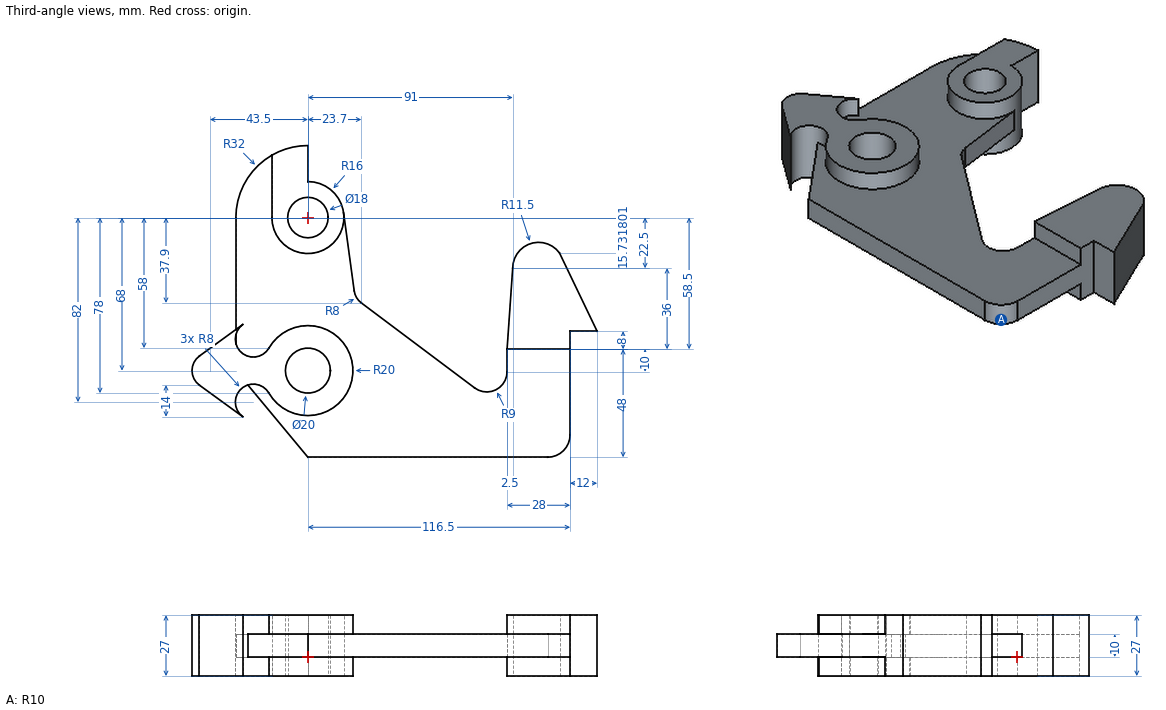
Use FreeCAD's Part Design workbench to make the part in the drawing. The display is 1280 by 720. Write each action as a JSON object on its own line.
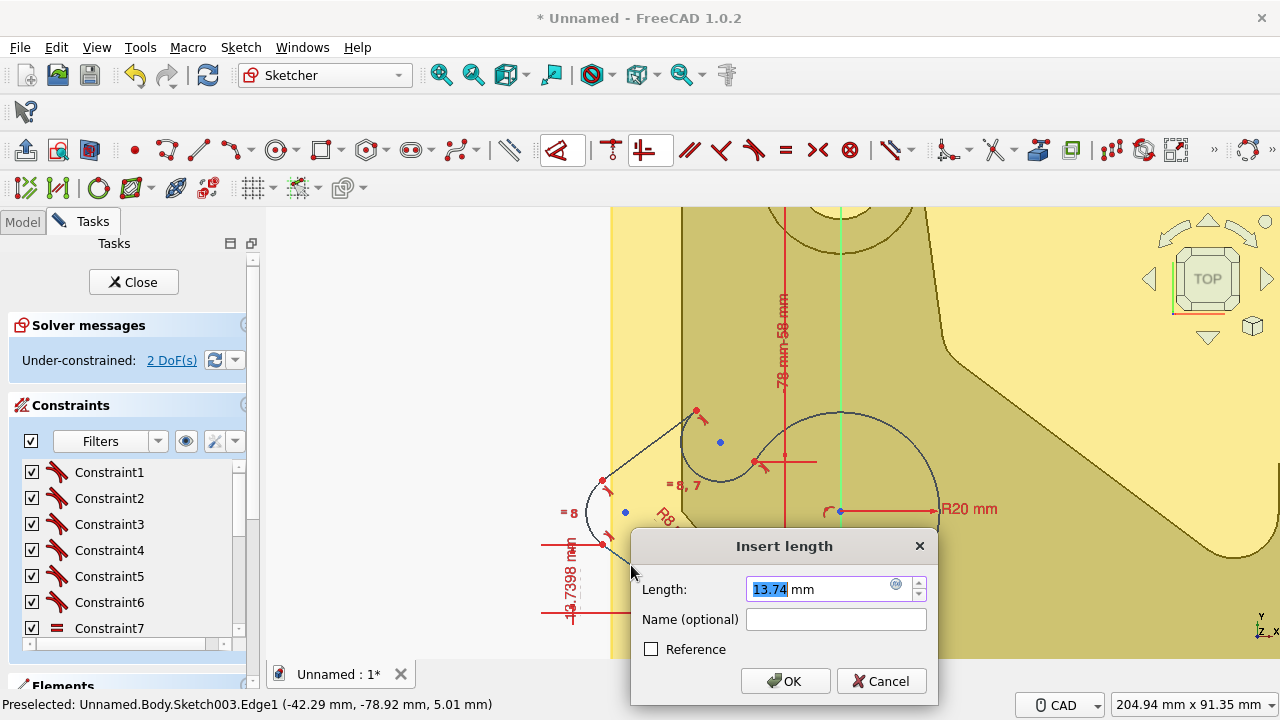
{"action": "type", "text": "14"}
{"action": "key", "text": "Return"}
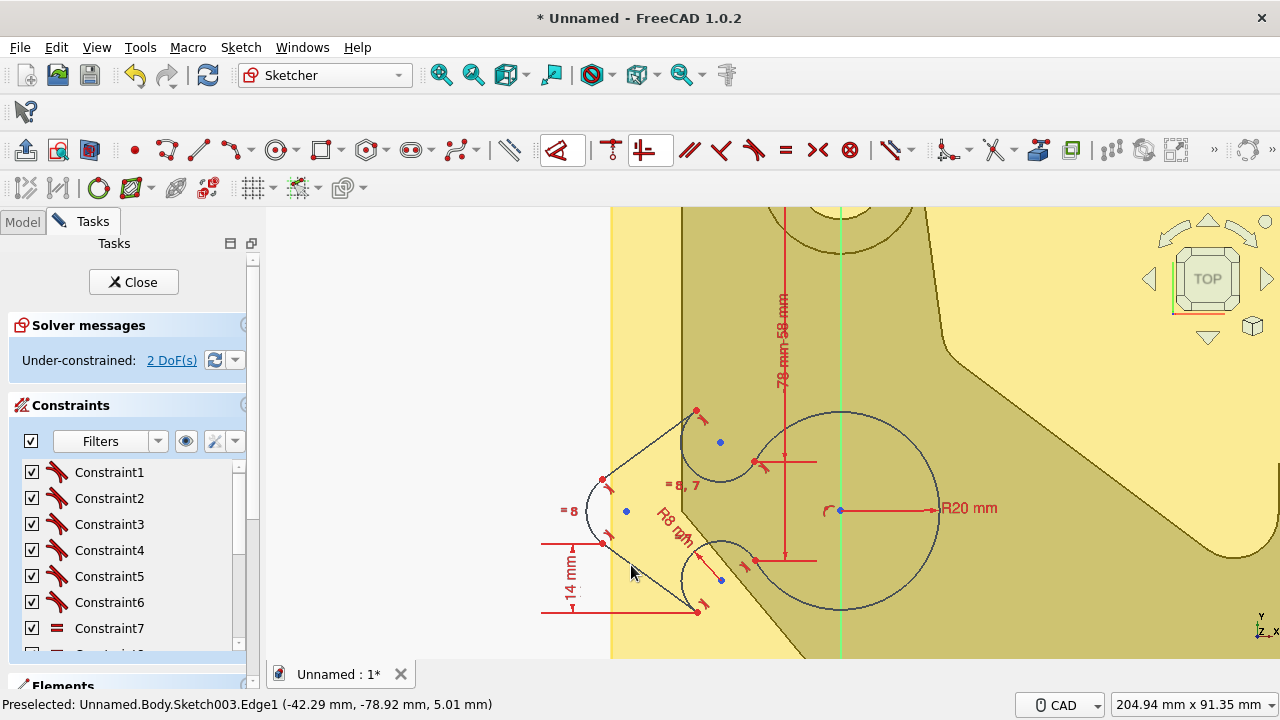
{"action": "left_click", "coordinate": [721, 581]}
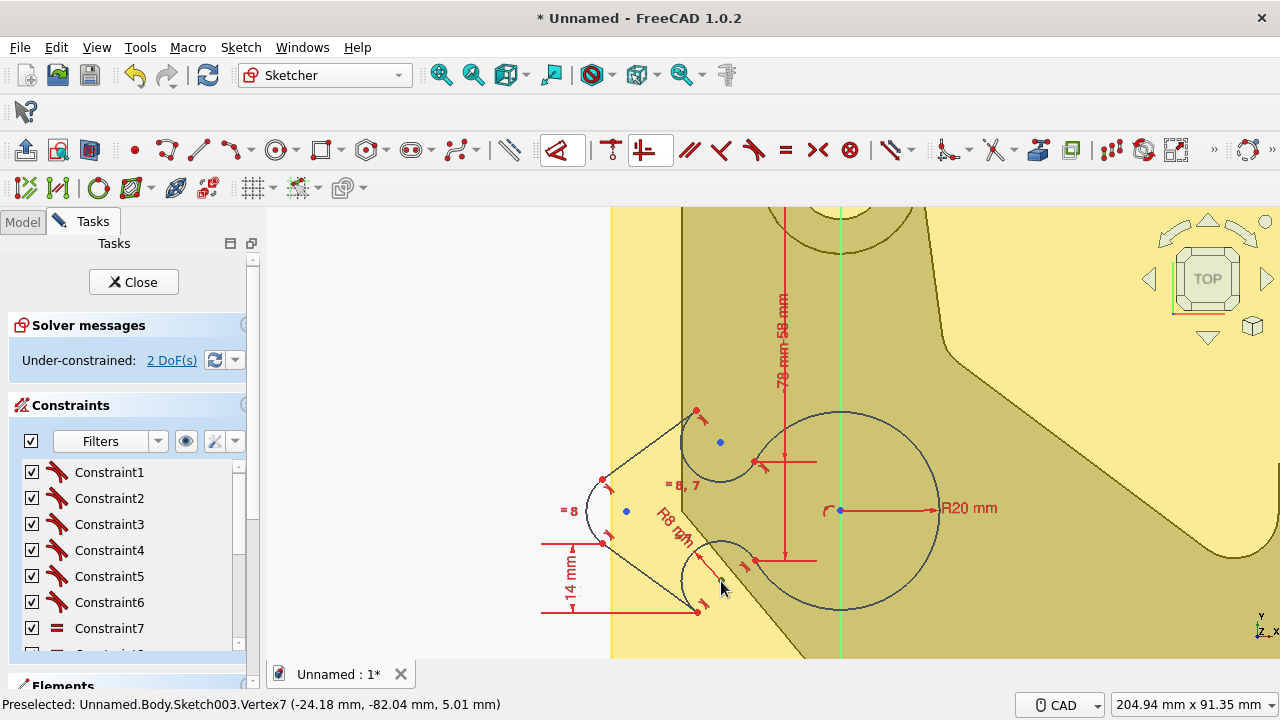
{"action": "left_click", "coordinate": [580, 150]}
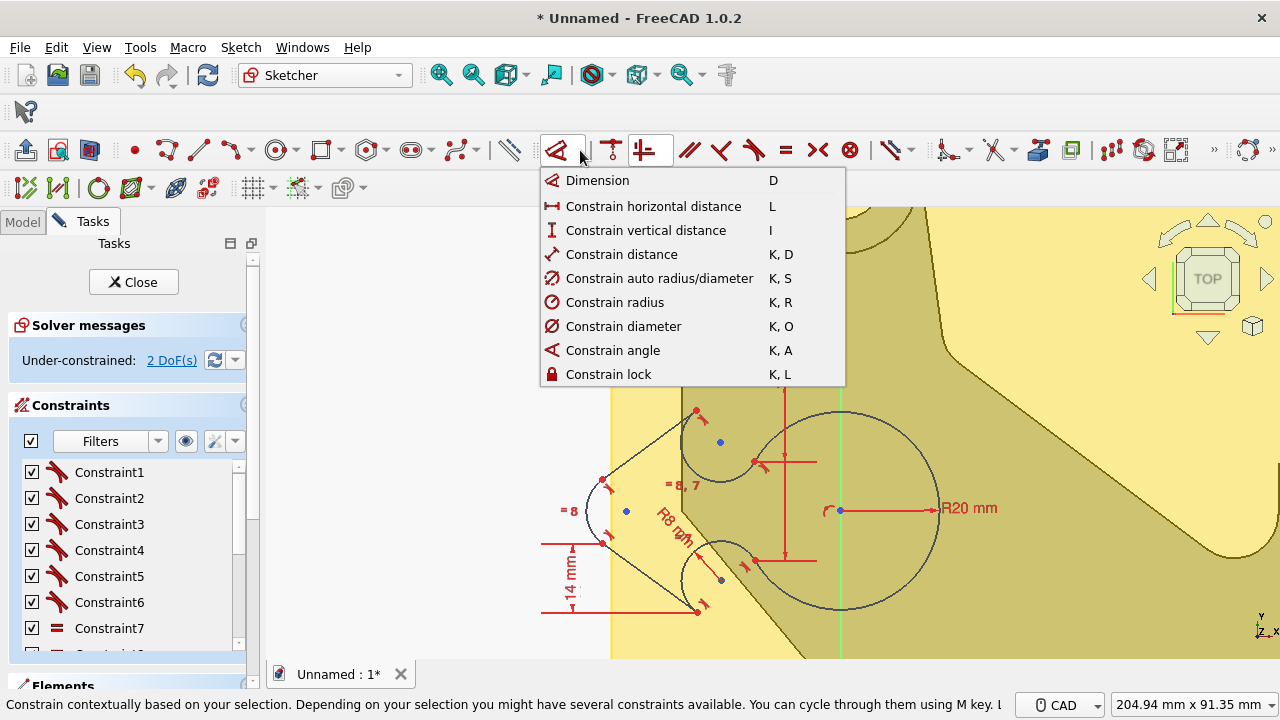
{"action": "left_click", "coordinate": [693, 230]}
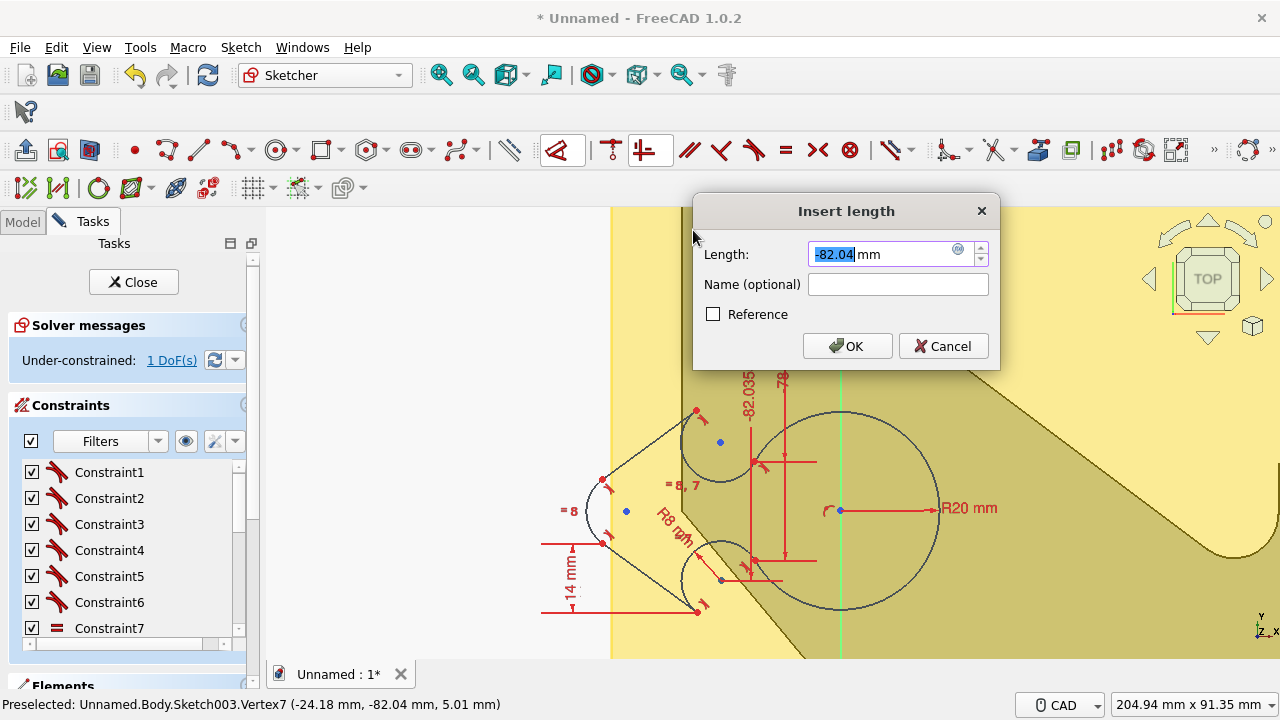
{"action": "type", "text": "-82"}
{"action": "key", "text": "Return"}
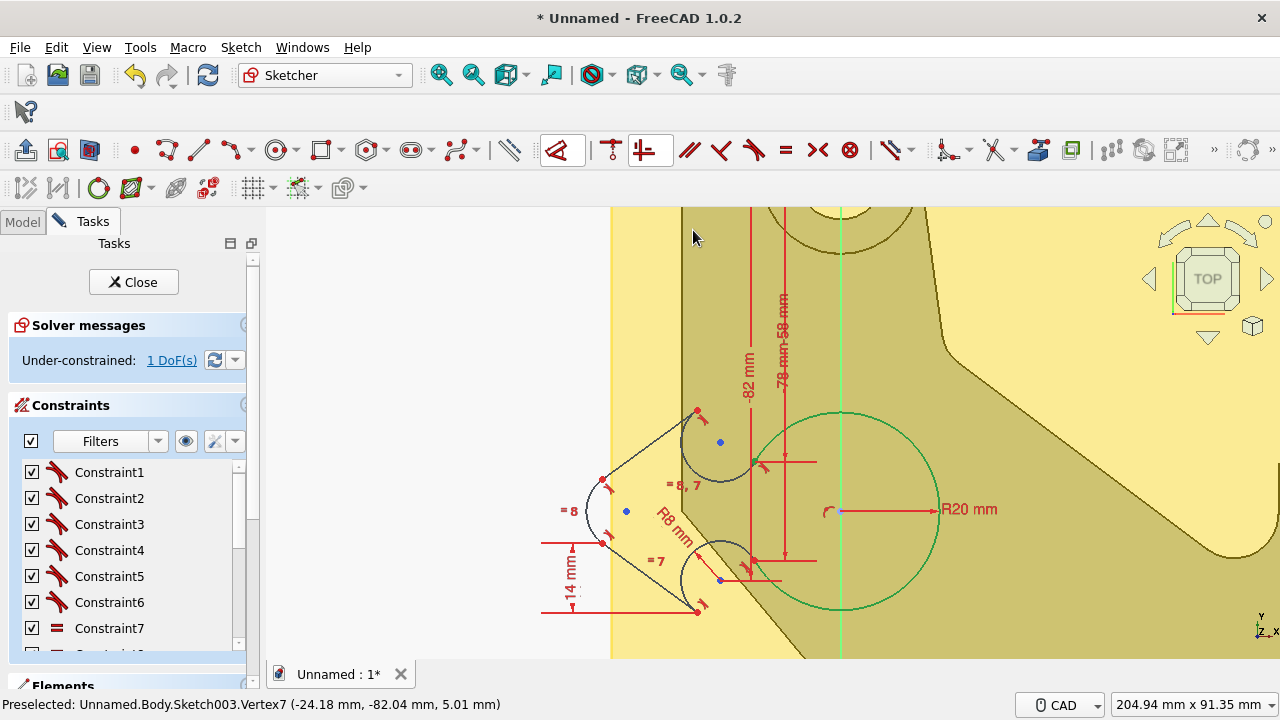
{"action": "left_click", "coordinate": [626, 511]}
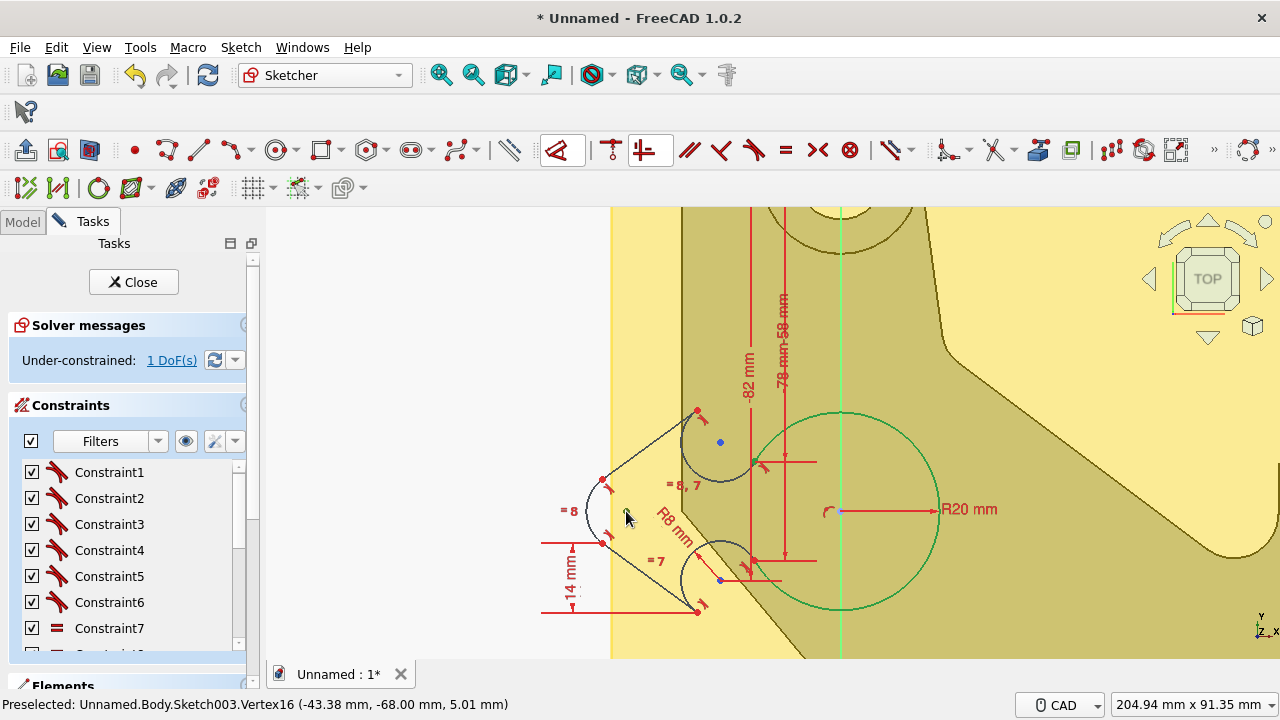
{"action": "key", "text": "l"}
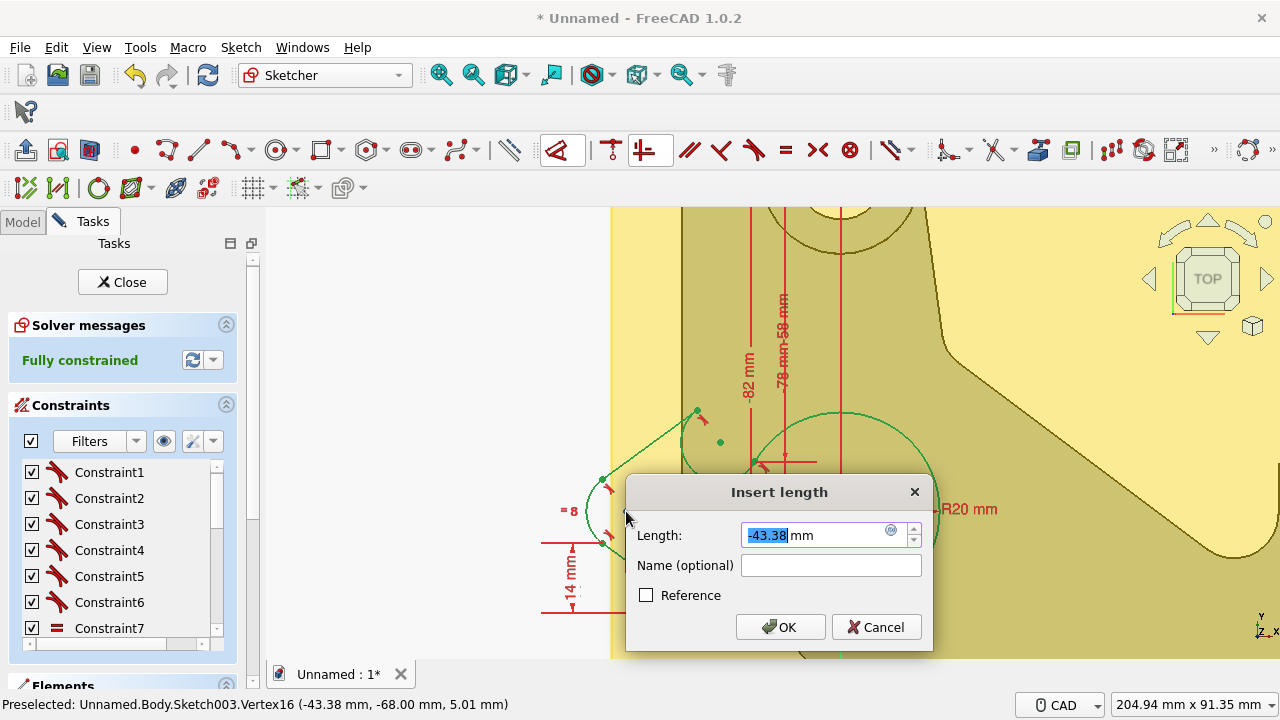
{"action": "type", "text": "-43.5"}
{"action": "key", "text": "Return"}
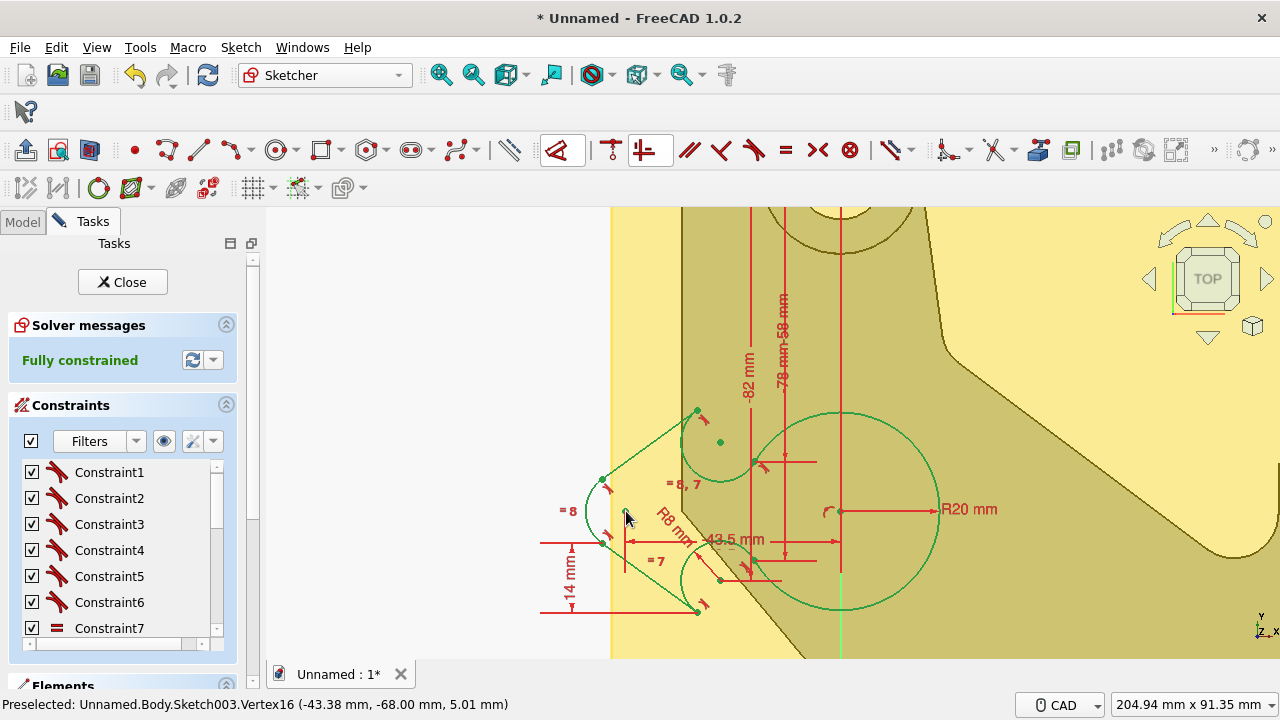
{"action": "left_click", "coordinate": [123, 282]}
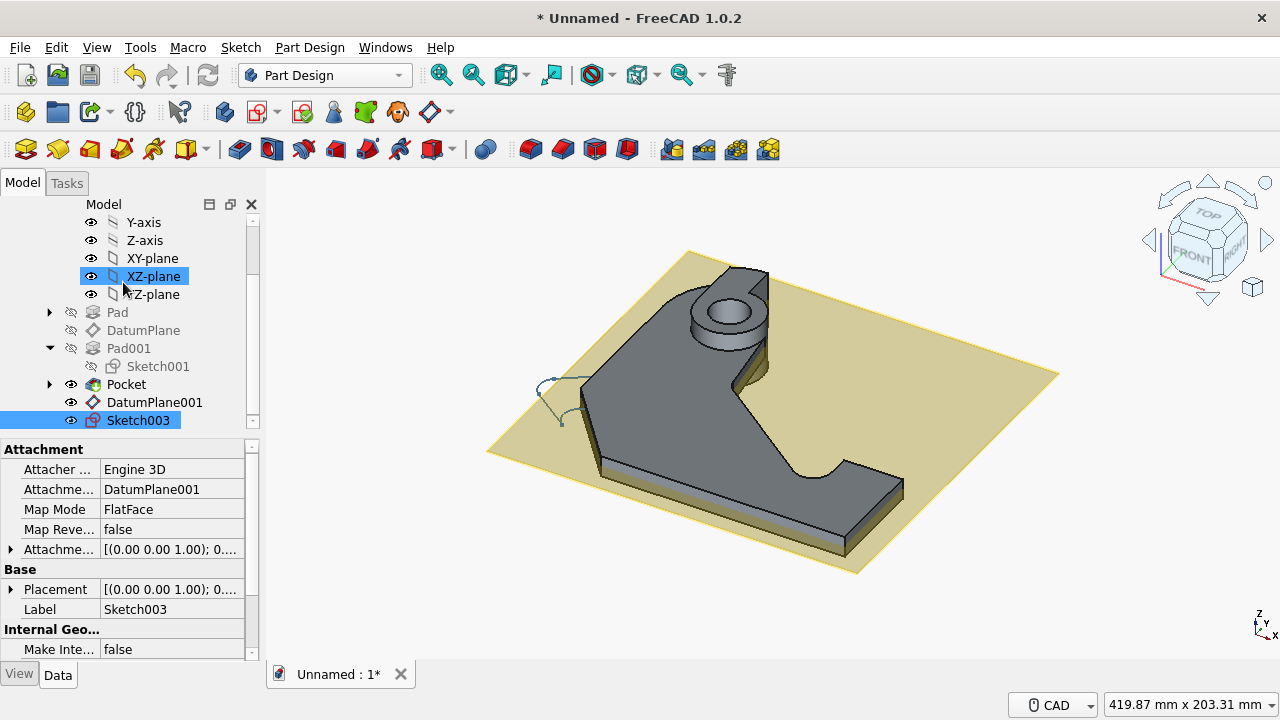
{"action": "left_click", "coordinate": [26, 150]}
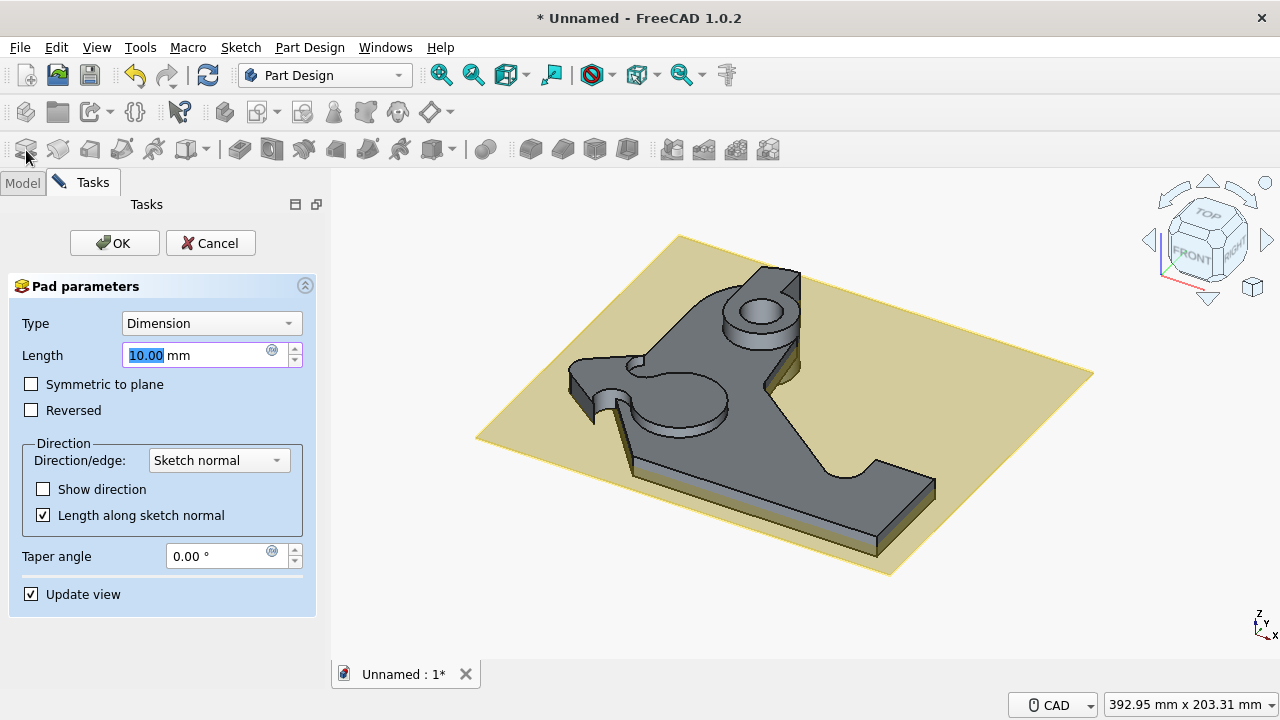
{"action": "type", "text": "27"}
{"action": "key", "text": "Tab"}